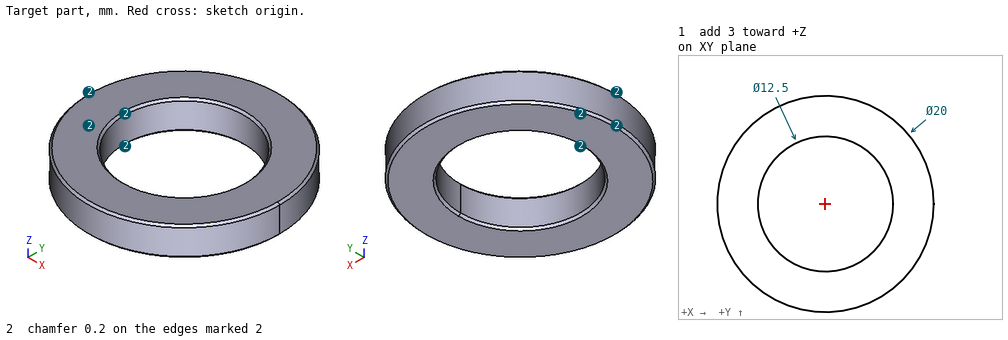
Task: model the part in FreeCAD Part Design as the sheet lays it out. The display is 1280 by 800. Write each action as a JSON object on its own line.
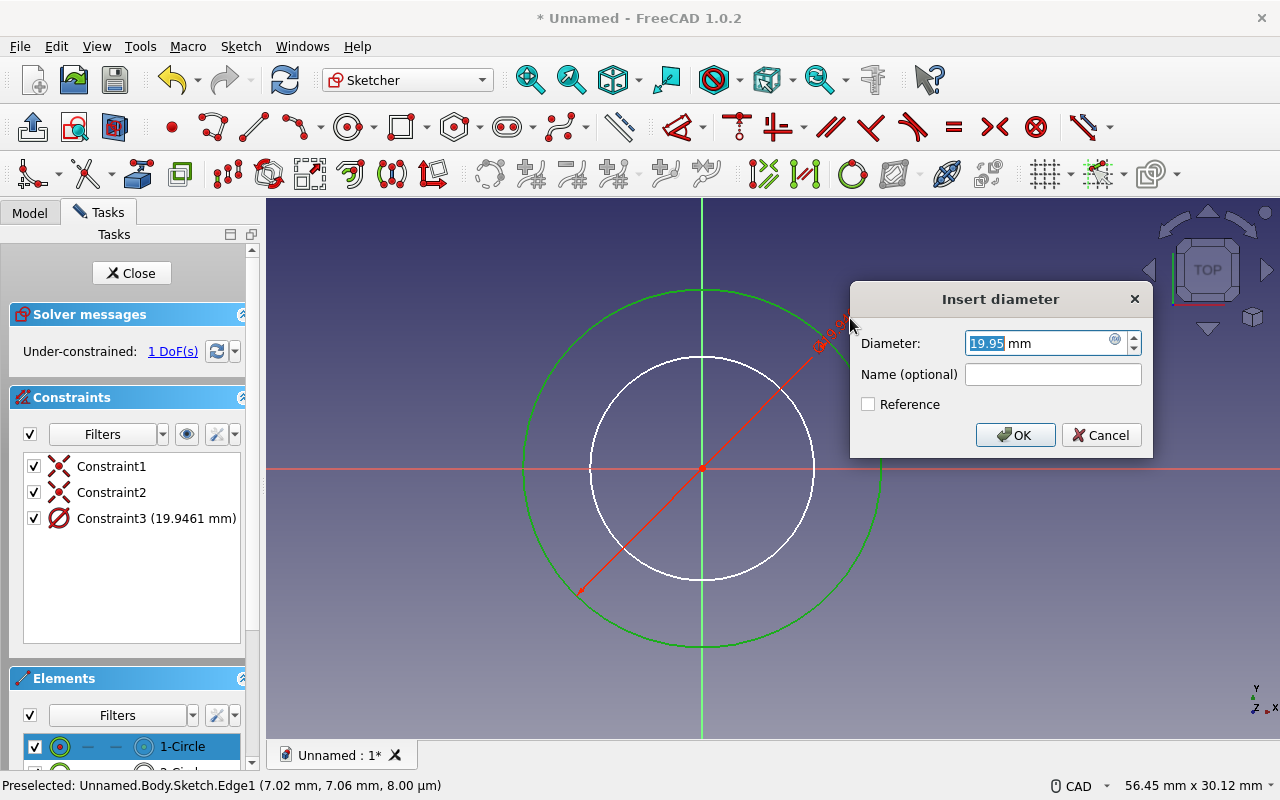
{"action": "type", "text": "20"}
{"action": "key", "text": "Return"}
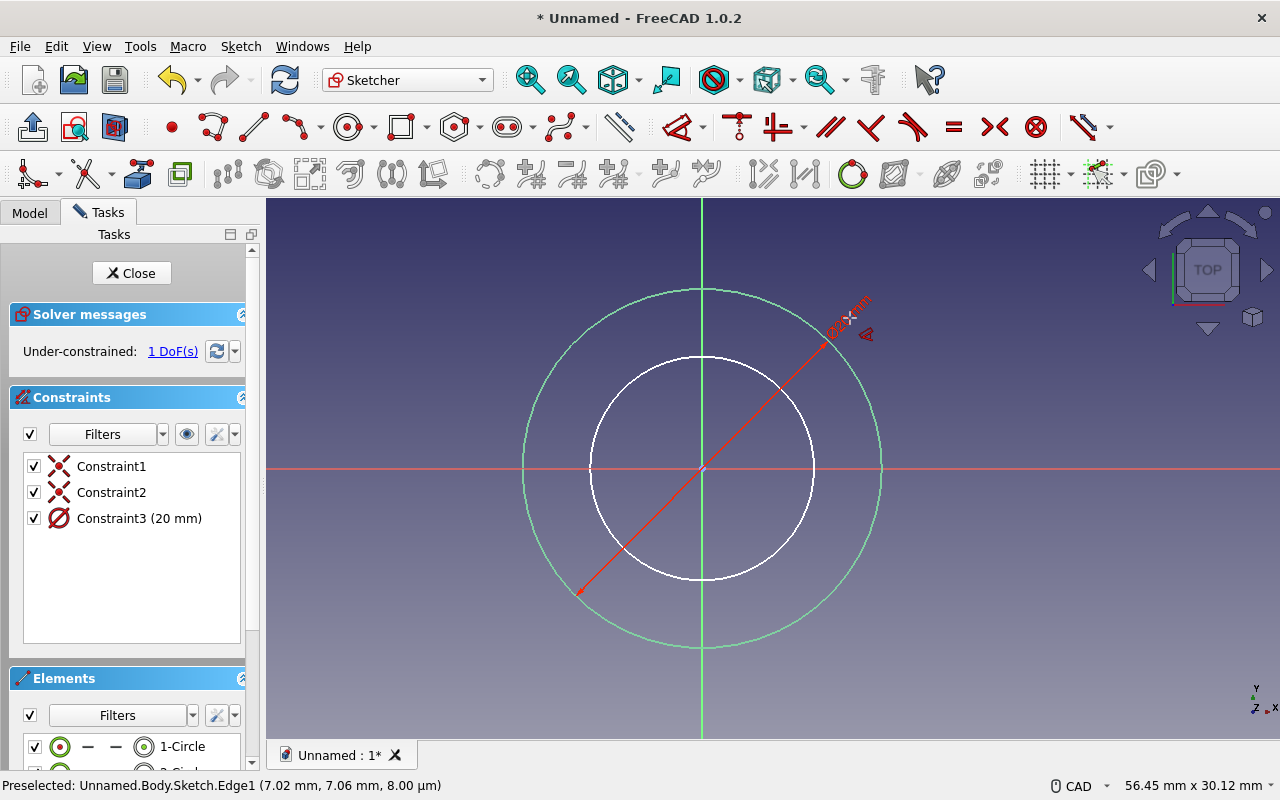
{"action": "left_click", "coordinate": [781, 389]}
{"action": "left_click", "coordinate": [804, 366]}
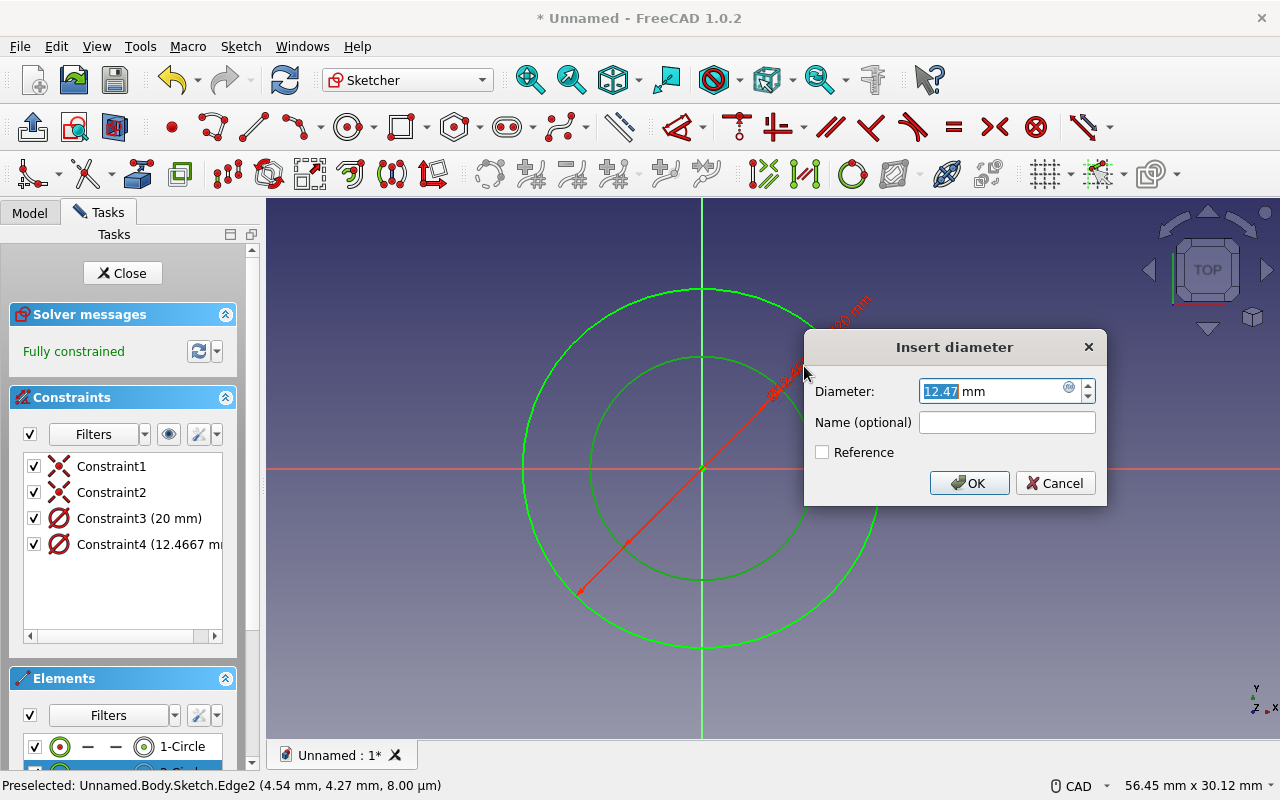
{"action": "type", "text": "12.5"}
{"action": "key", "text": "Return"}
{"action": "key", "text": "Escape"}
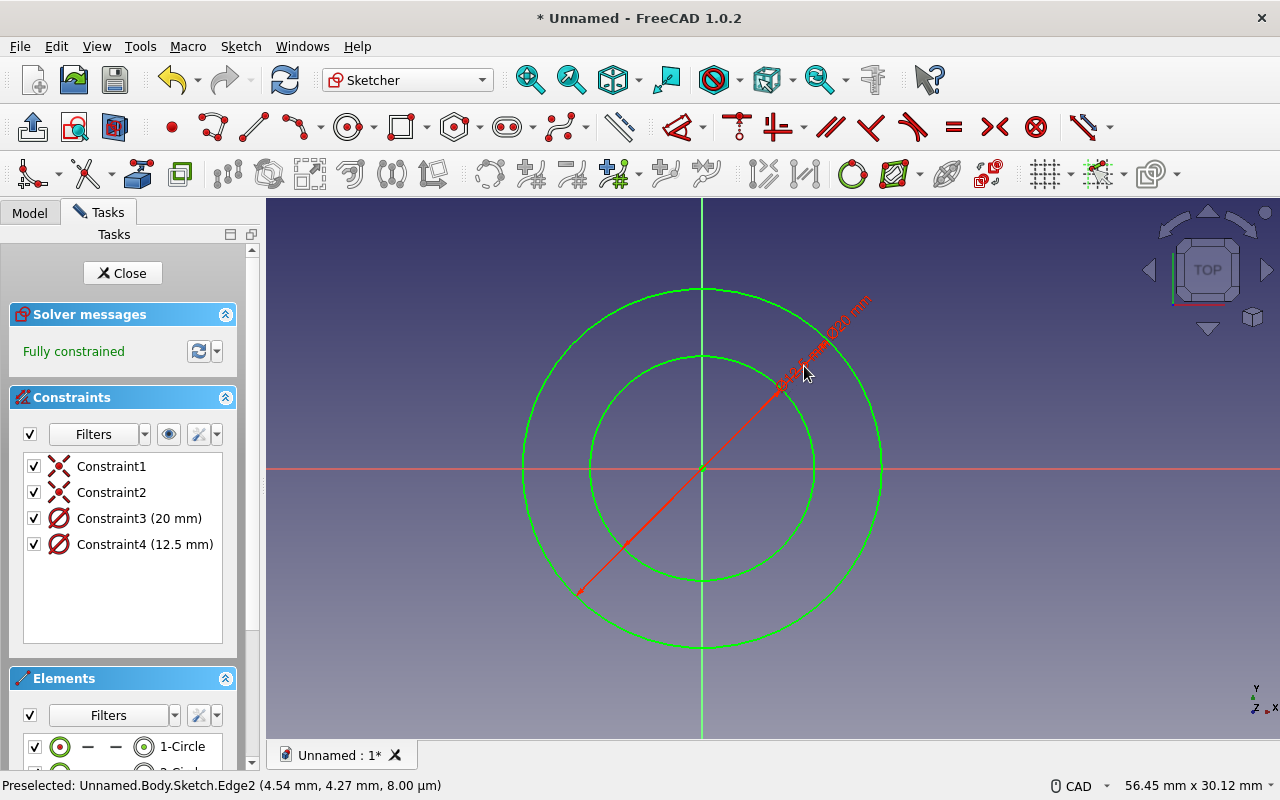
{"action": "left_click", "coordinate": [123, 273]}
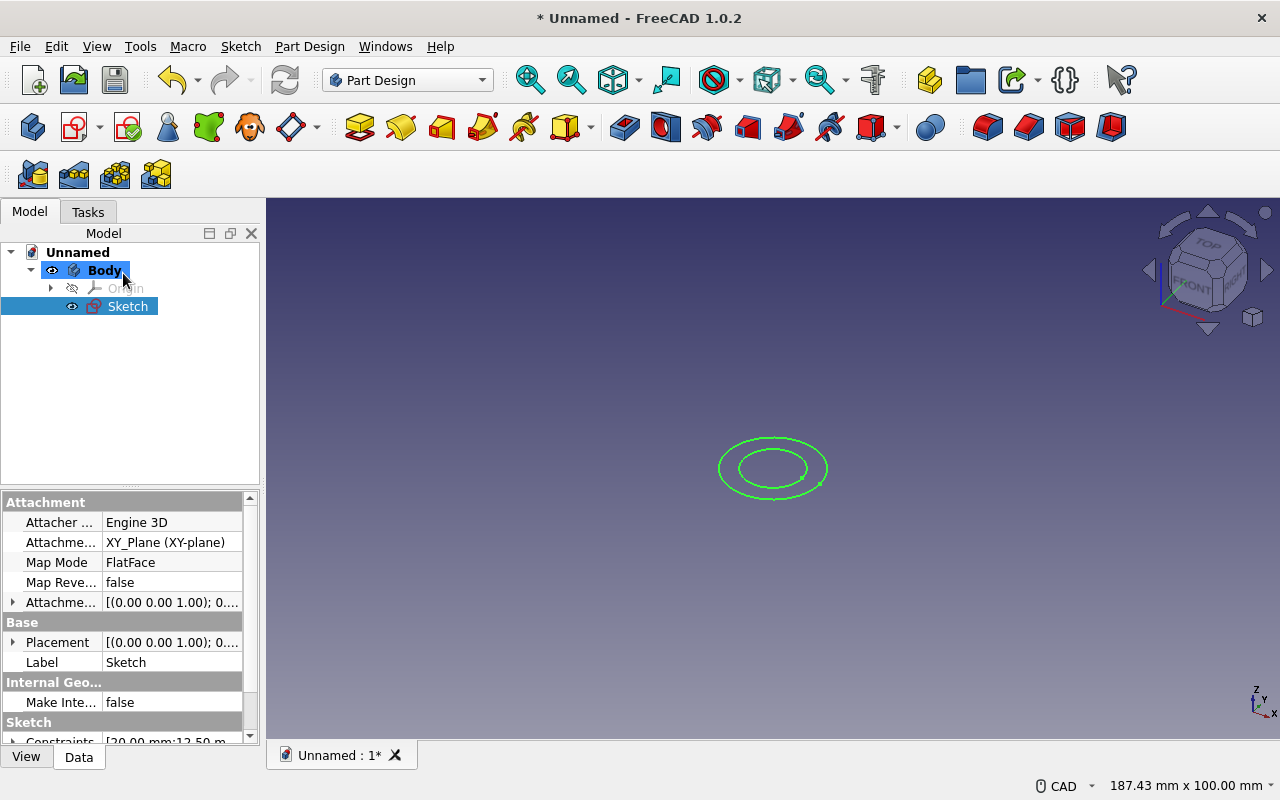
{"action": "left_click", "coordinate": [360, 128]}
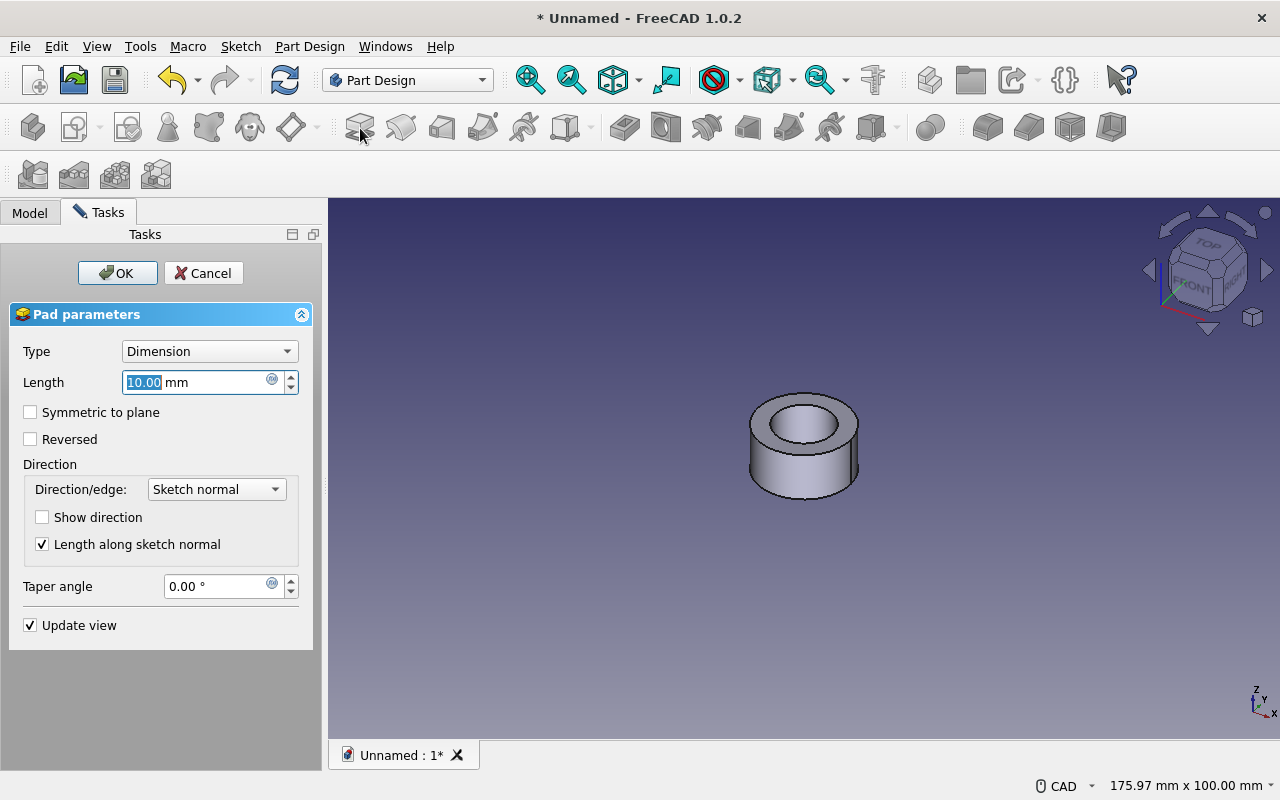
{"action": "type", "text": "3"}
{"action": "key", "text": "Tab"}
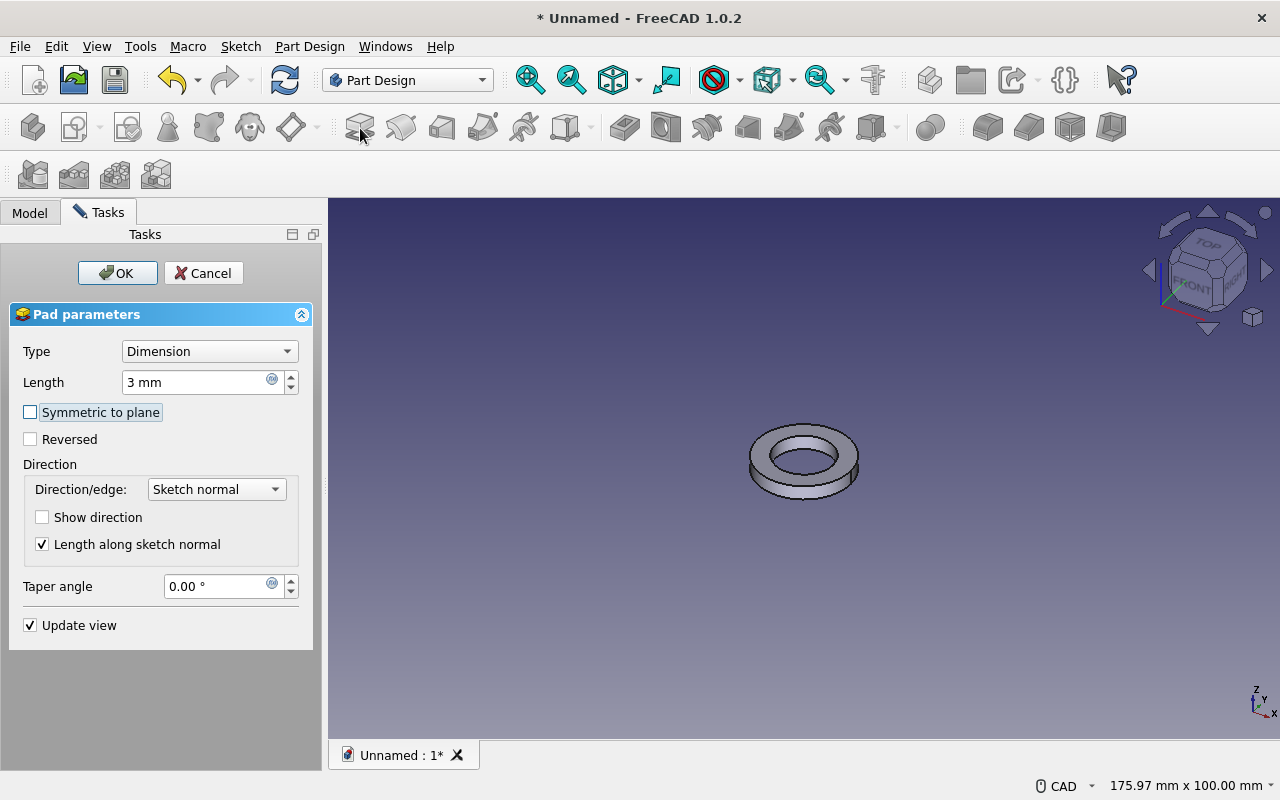
{"action": "left_click", "coordinate": [118, 273]}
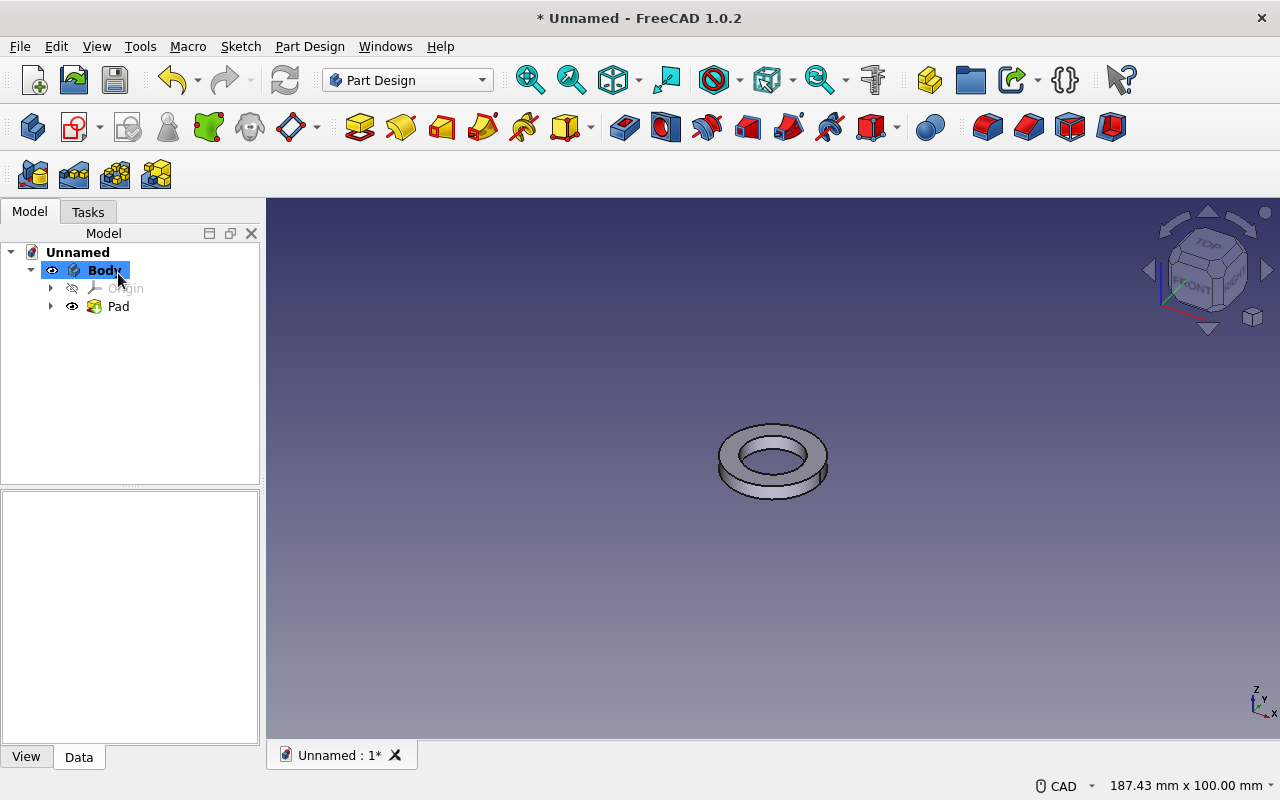
{"action": "left_click", "coordinate": [531, 80]}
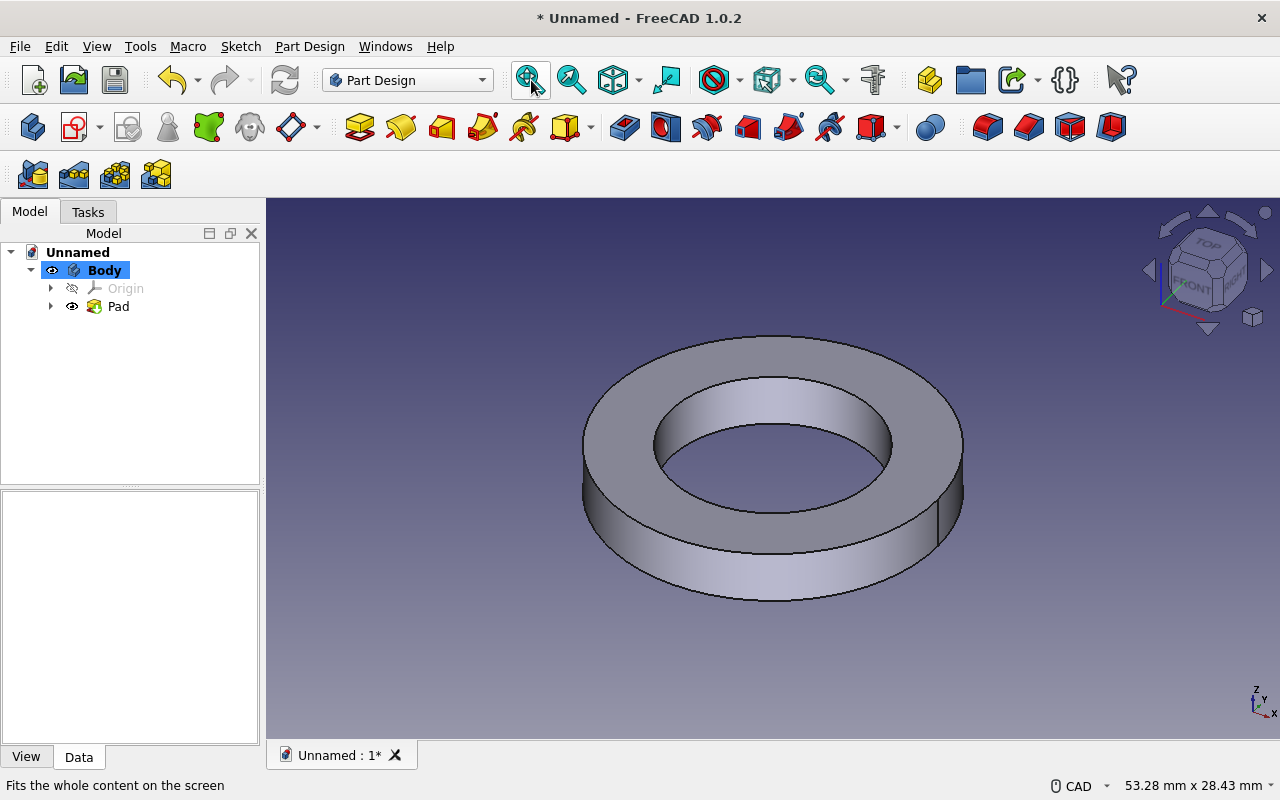
{"action": "left_click", "coordinate": [584, 455]}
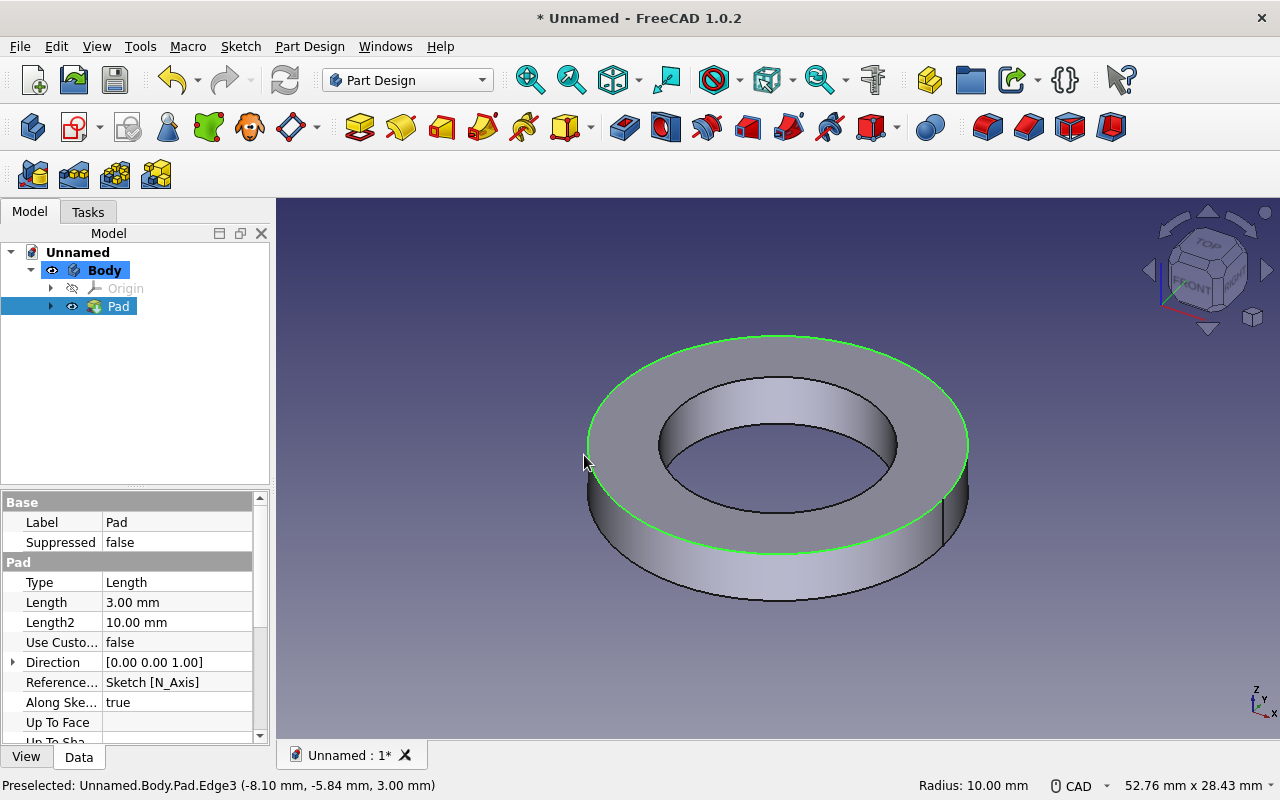
{"action": "left_click", "coordinate": [730, 429], "text": "ctrl"}